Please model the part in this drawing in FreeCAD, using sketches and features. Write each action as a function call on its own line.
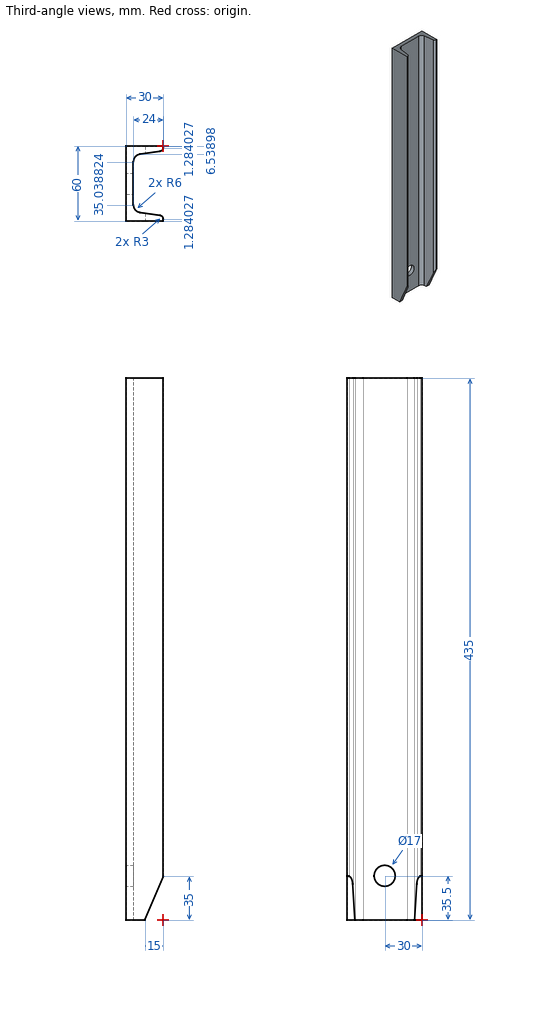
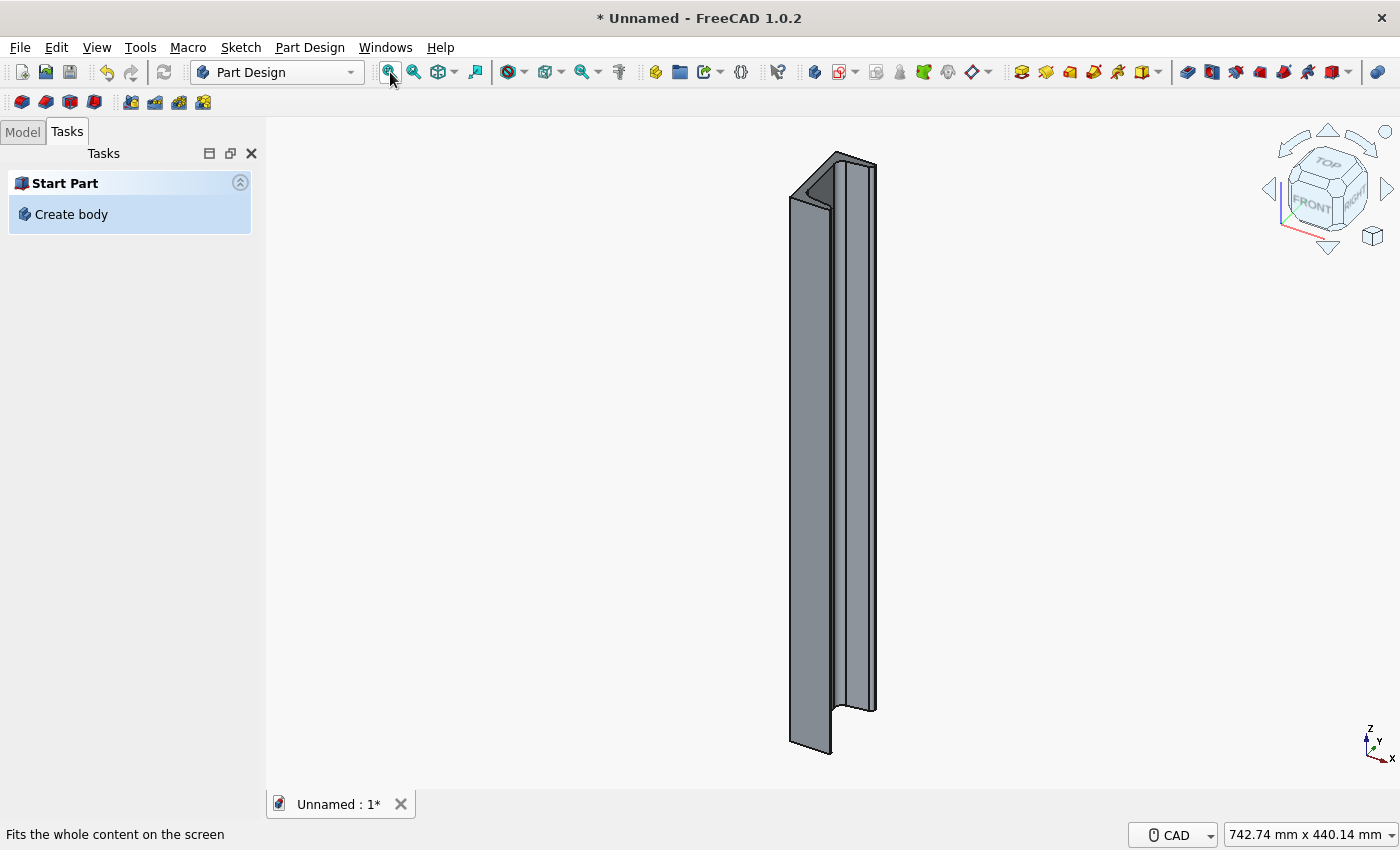
key(6)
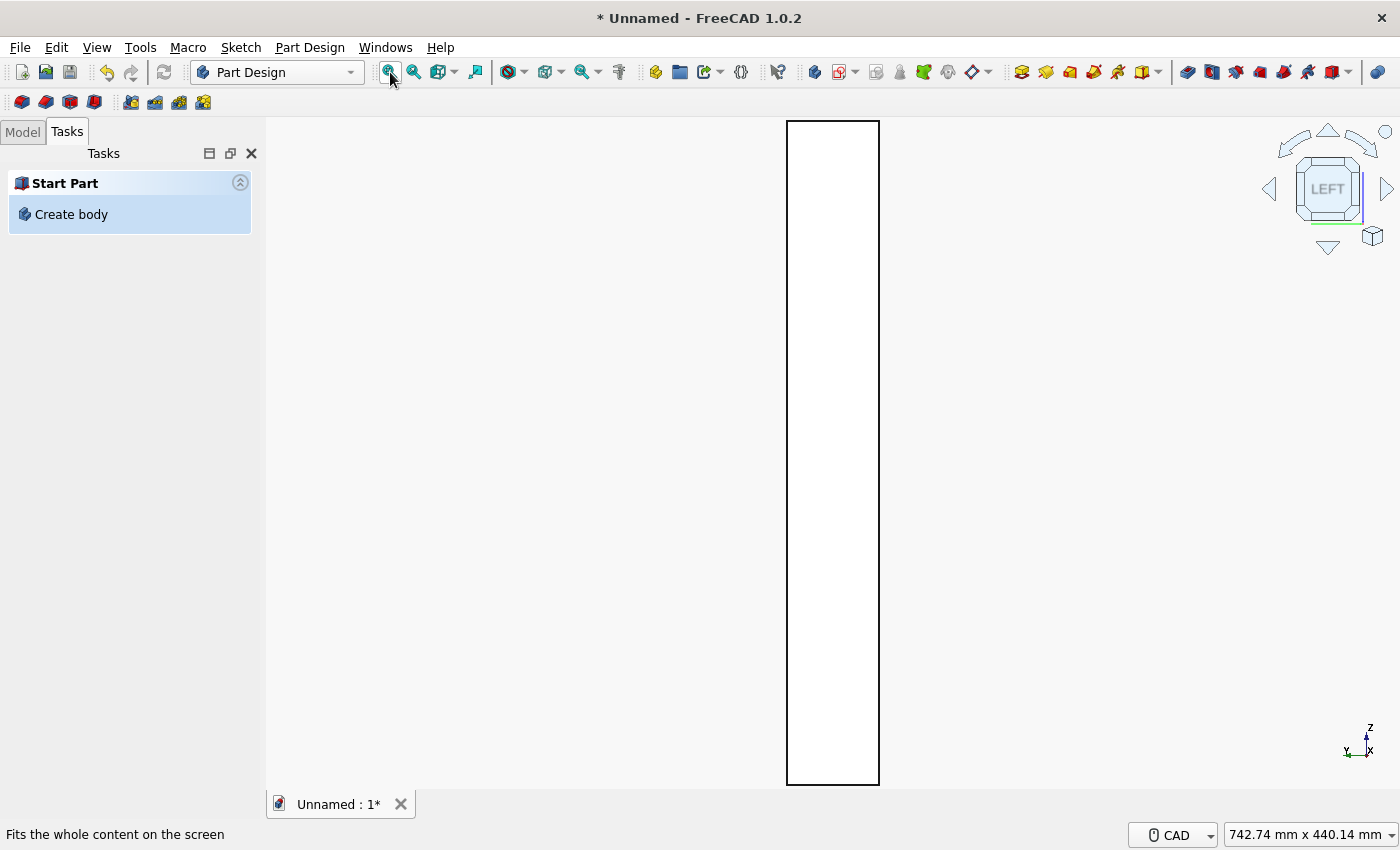
click(833, 167)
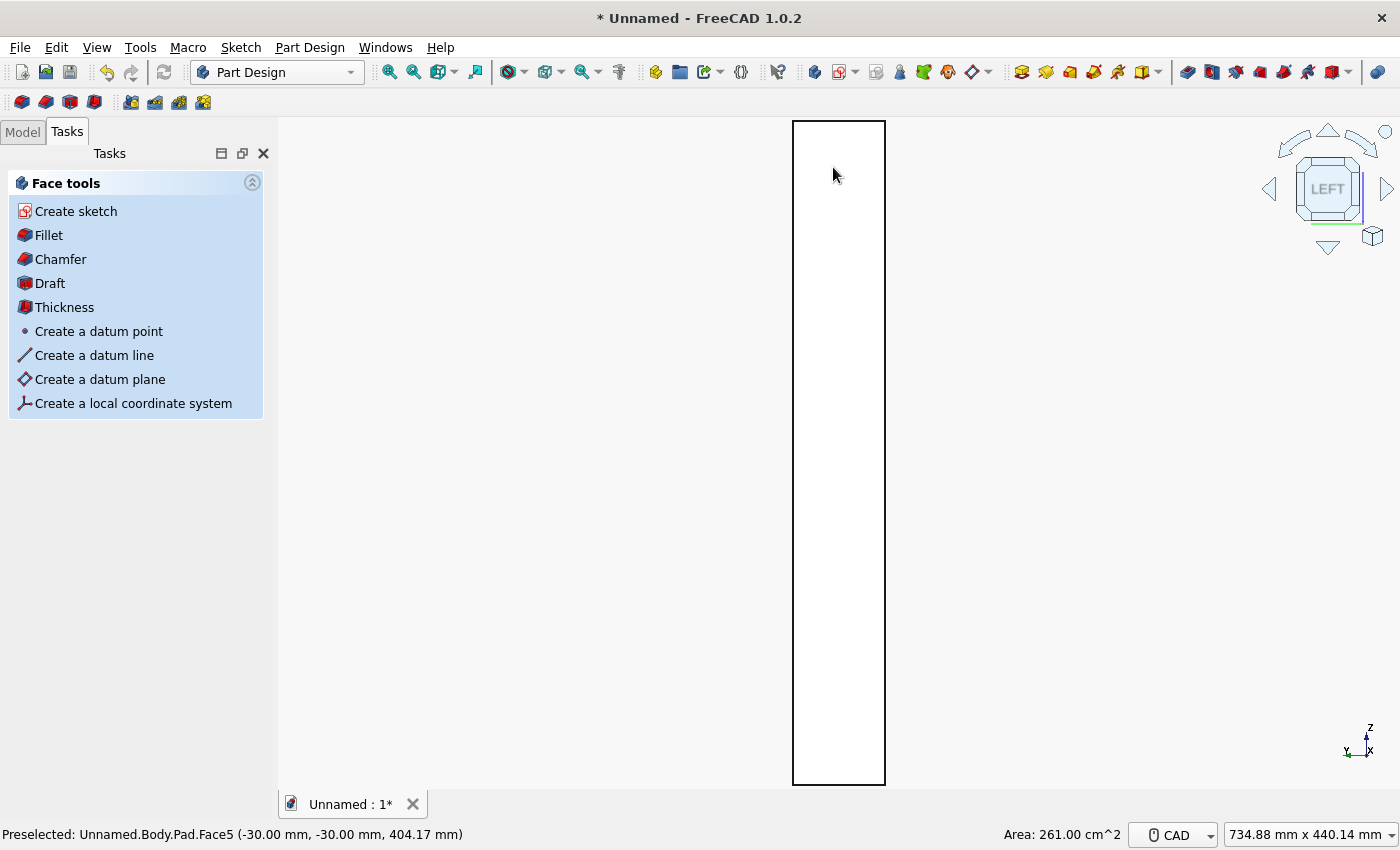
click(840, 72)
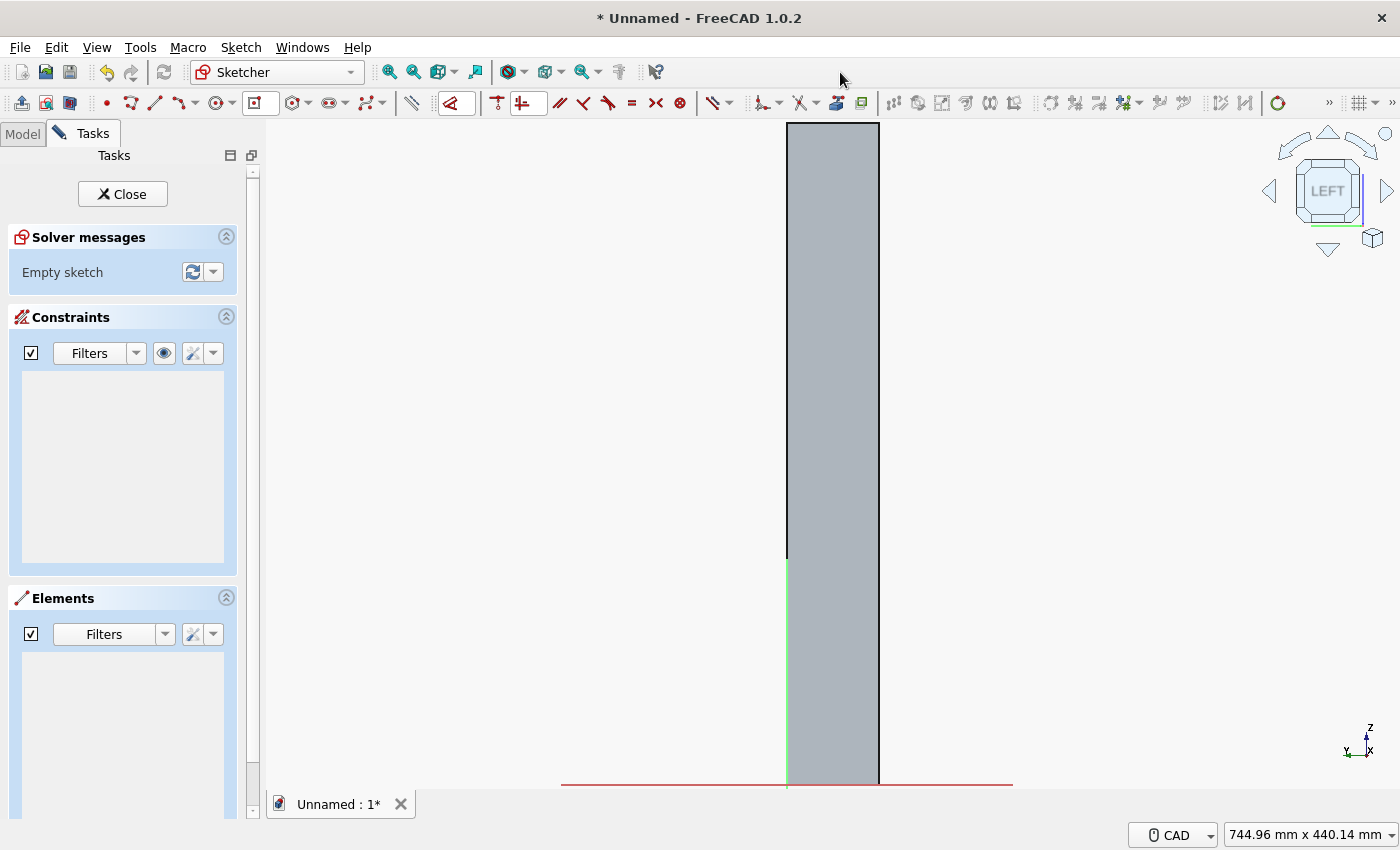
scroll(837, 749, up, 14)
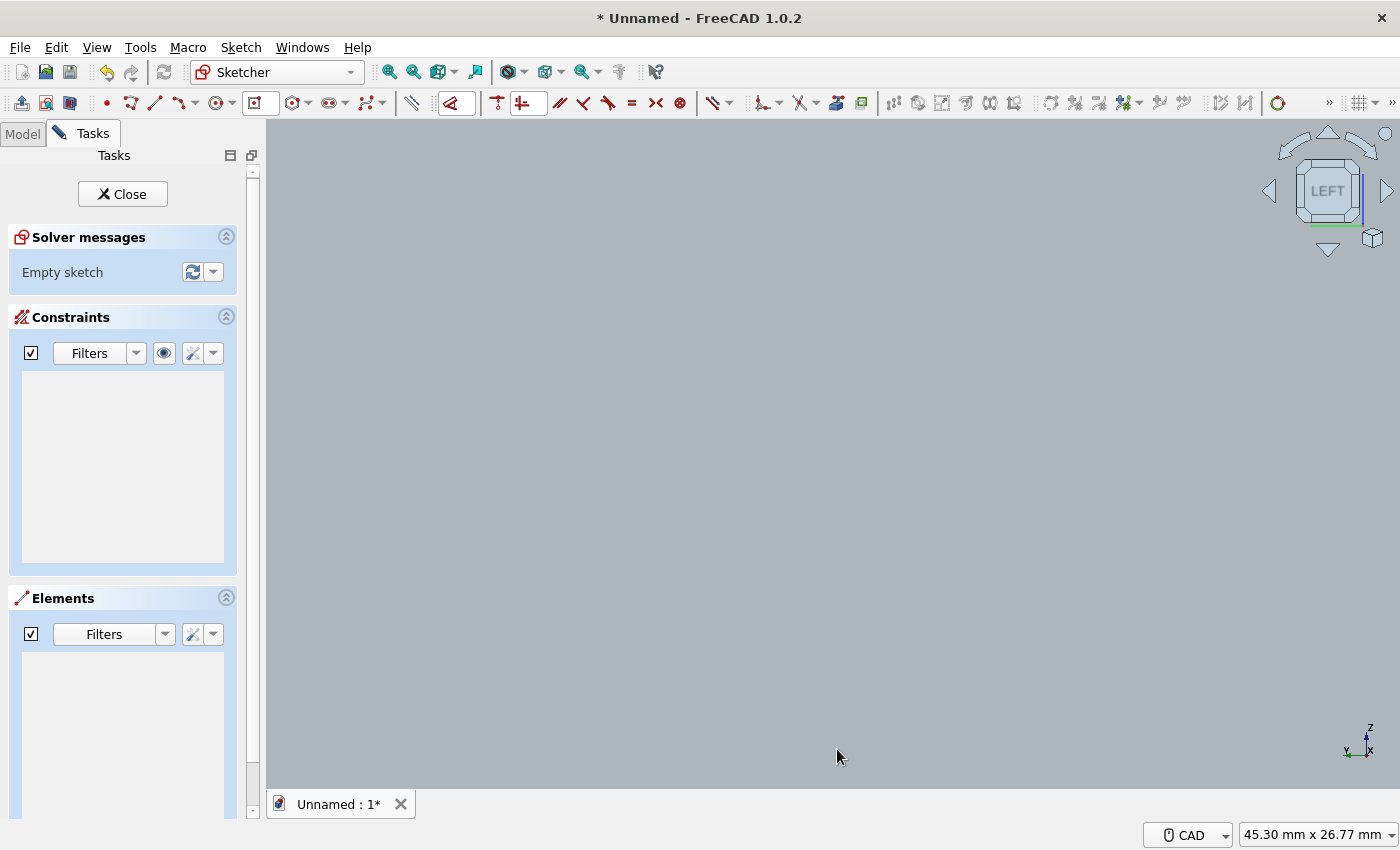
click(216, 104)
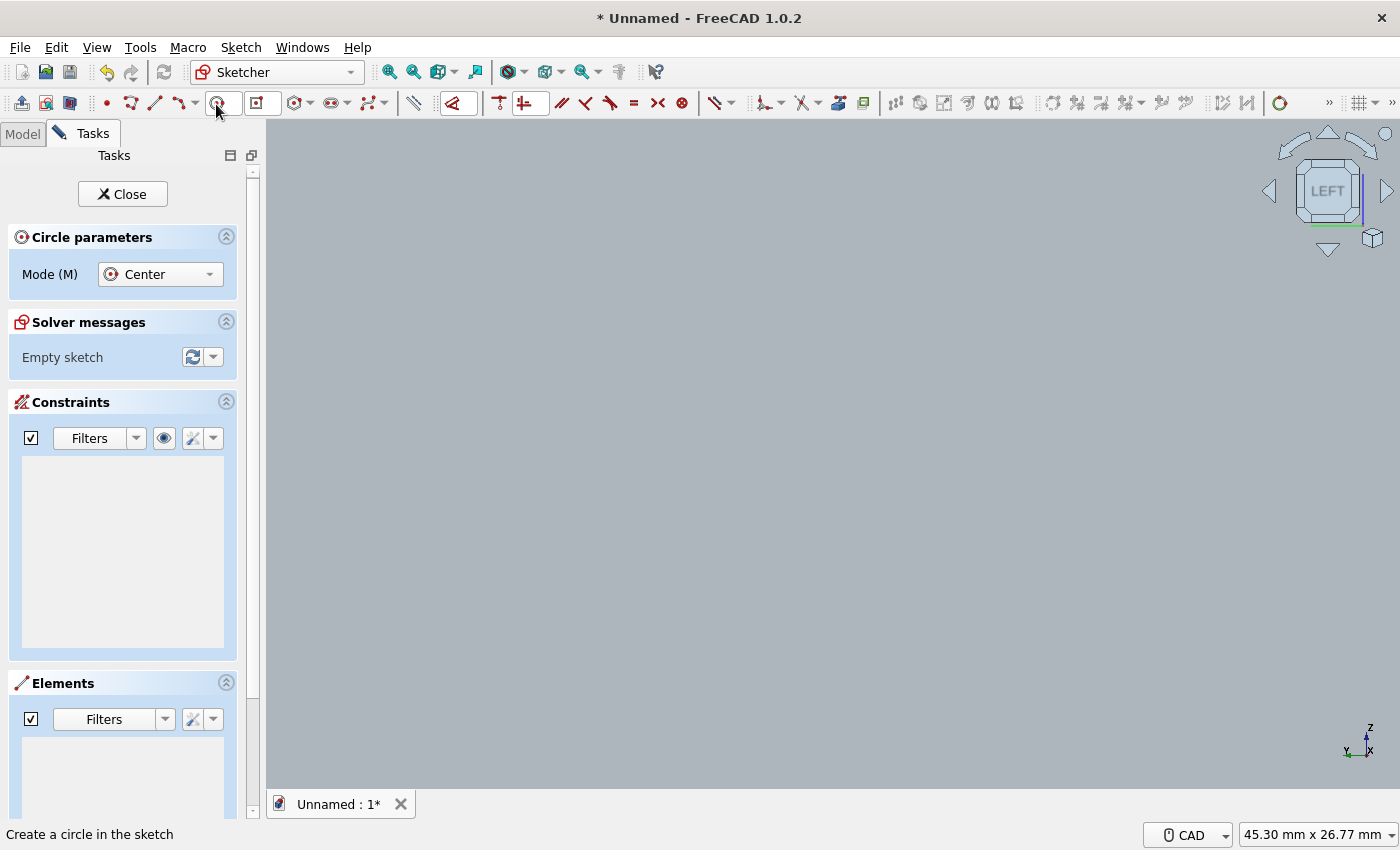
click(763, 439)
click(914, 289)
key(Escape)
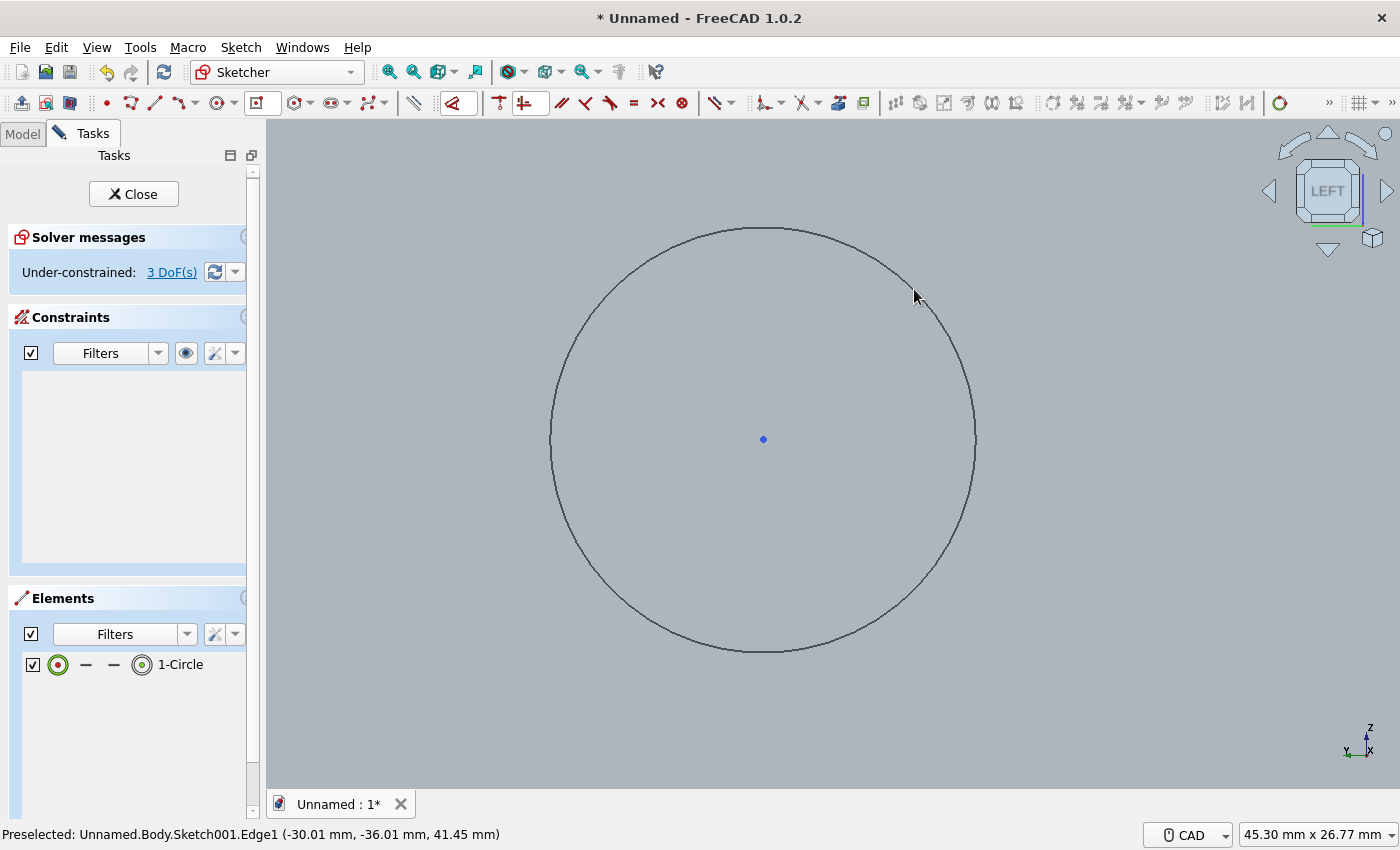
click(913, 289)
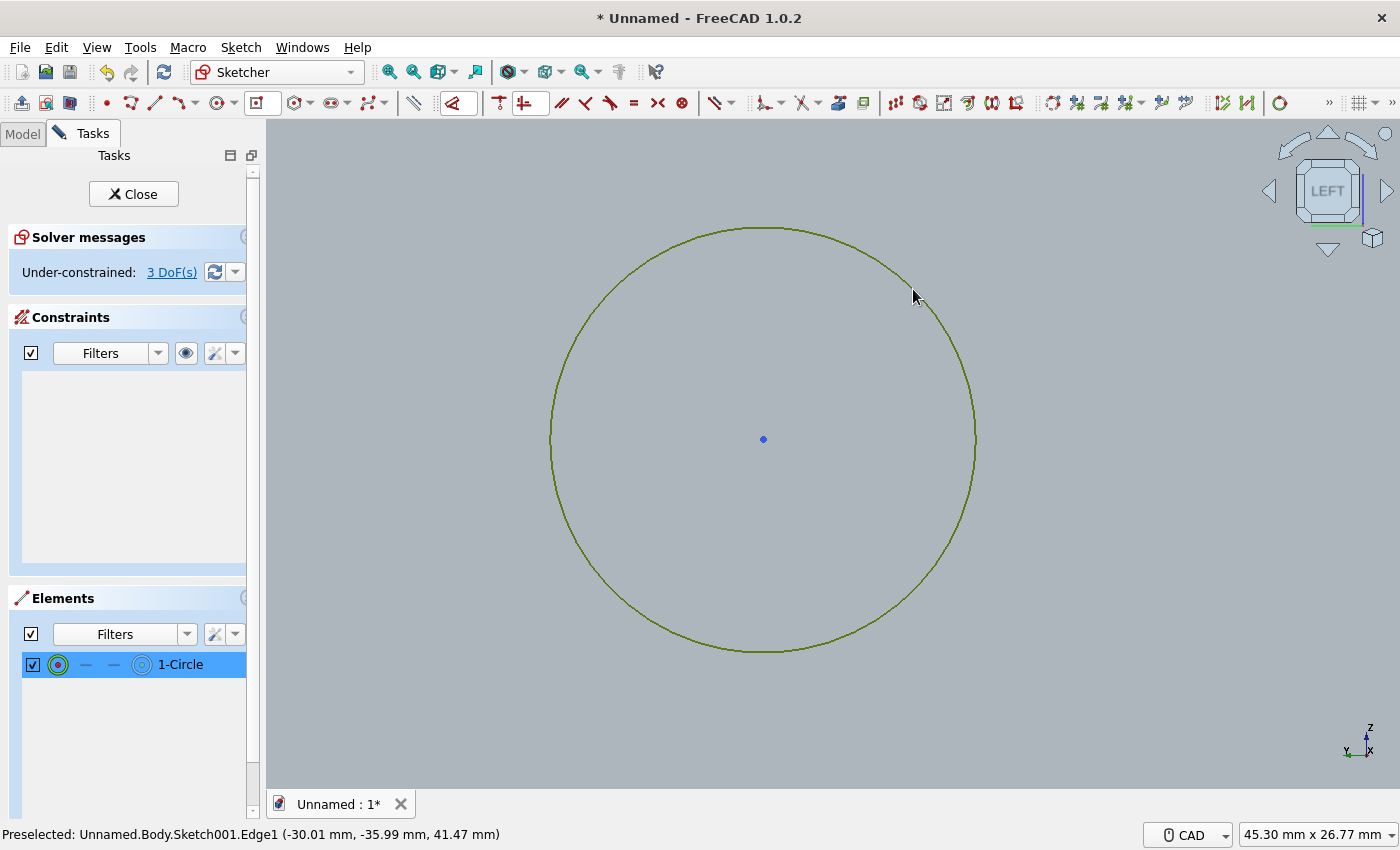
key(k)
key(o)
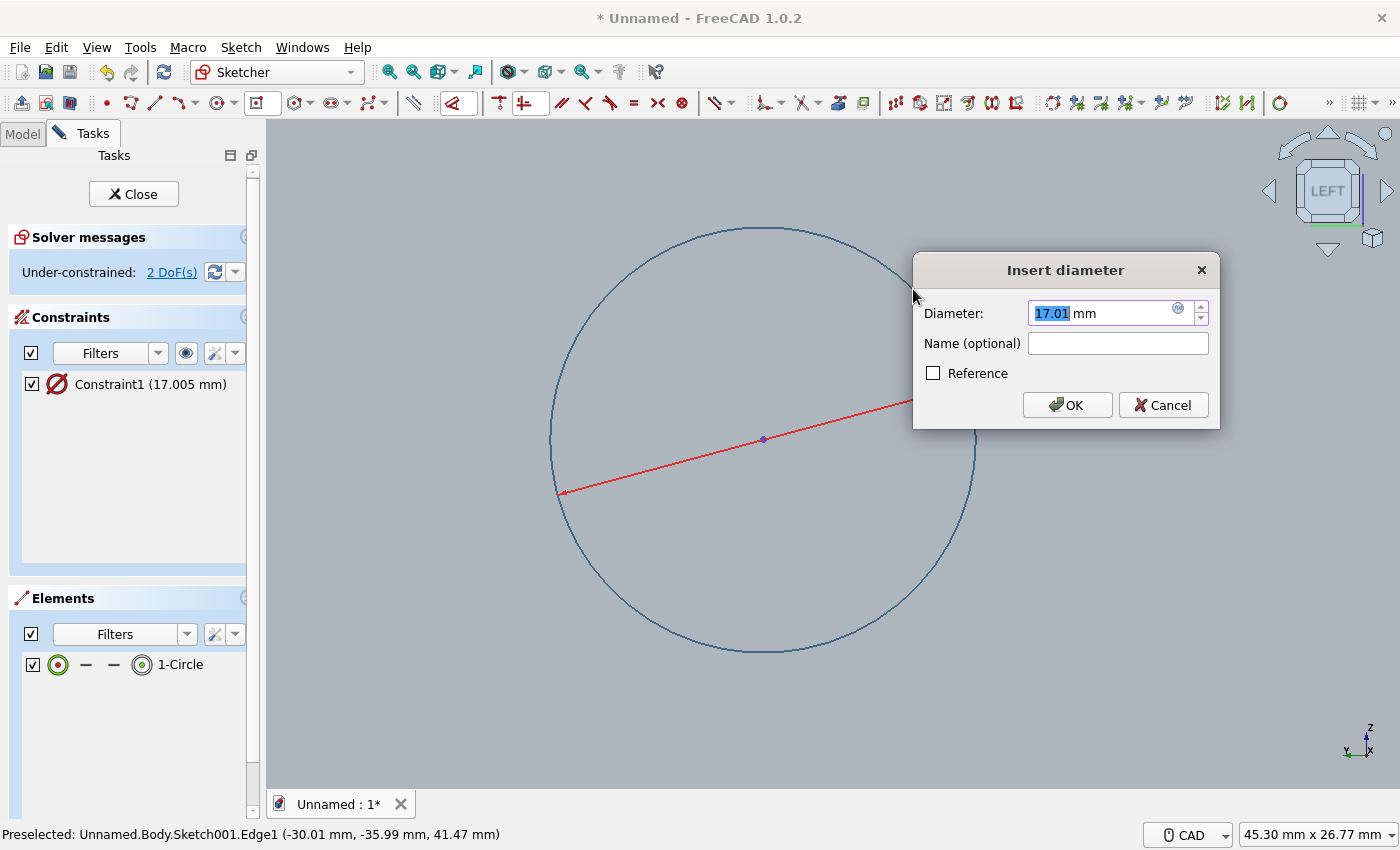
text(17)
key(Return)